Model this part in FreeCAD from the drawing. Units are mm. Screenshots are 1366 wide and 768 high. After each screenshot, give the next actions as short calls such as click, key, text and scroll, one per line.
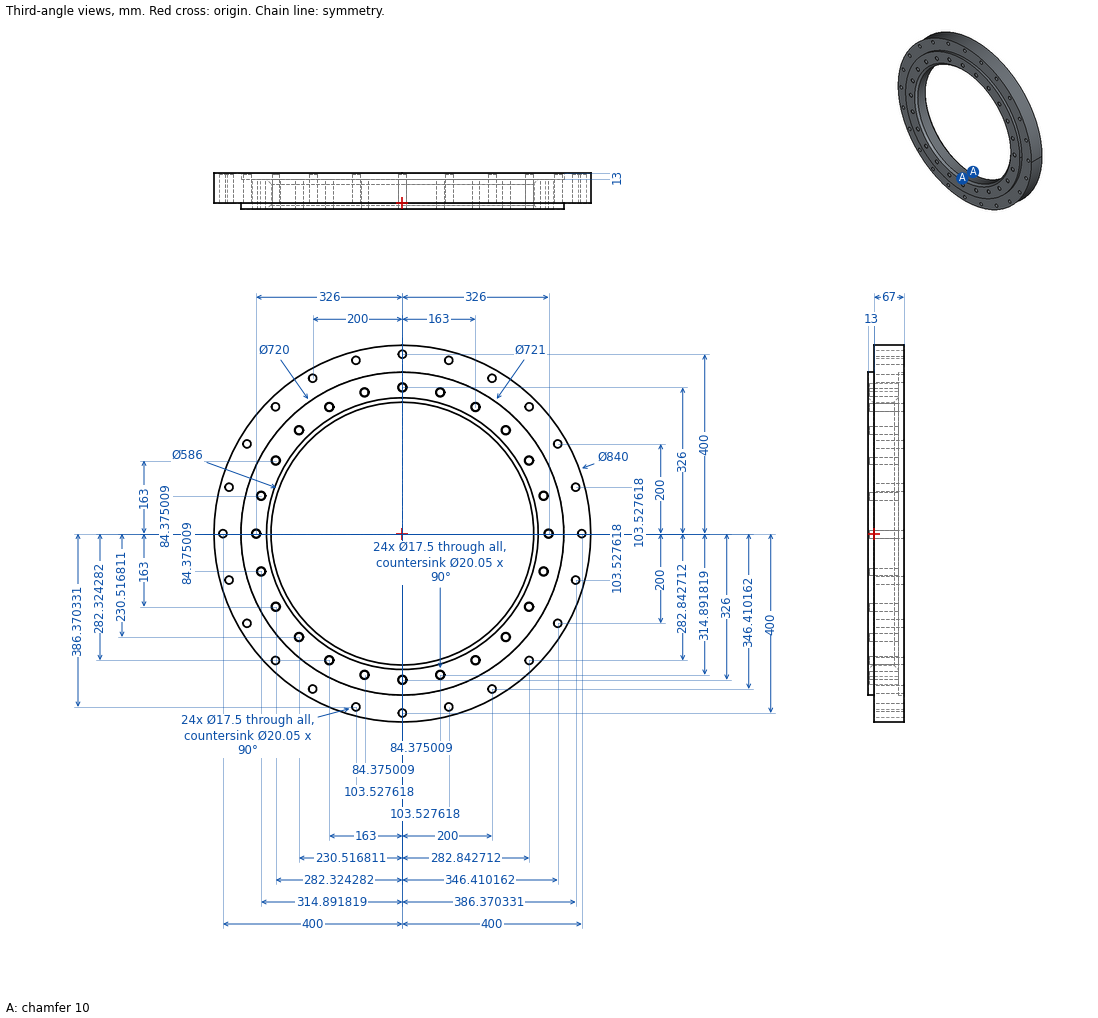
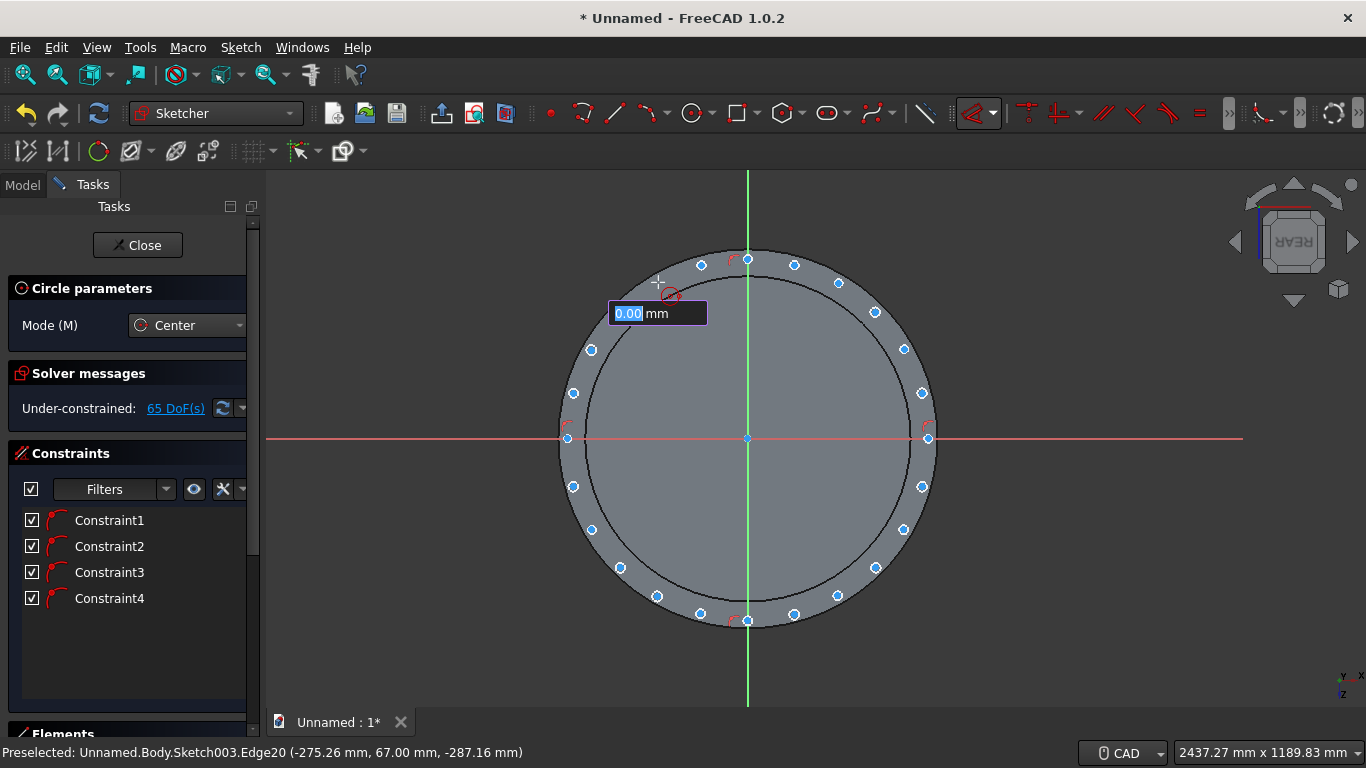
scroll(660, 280, up, 7)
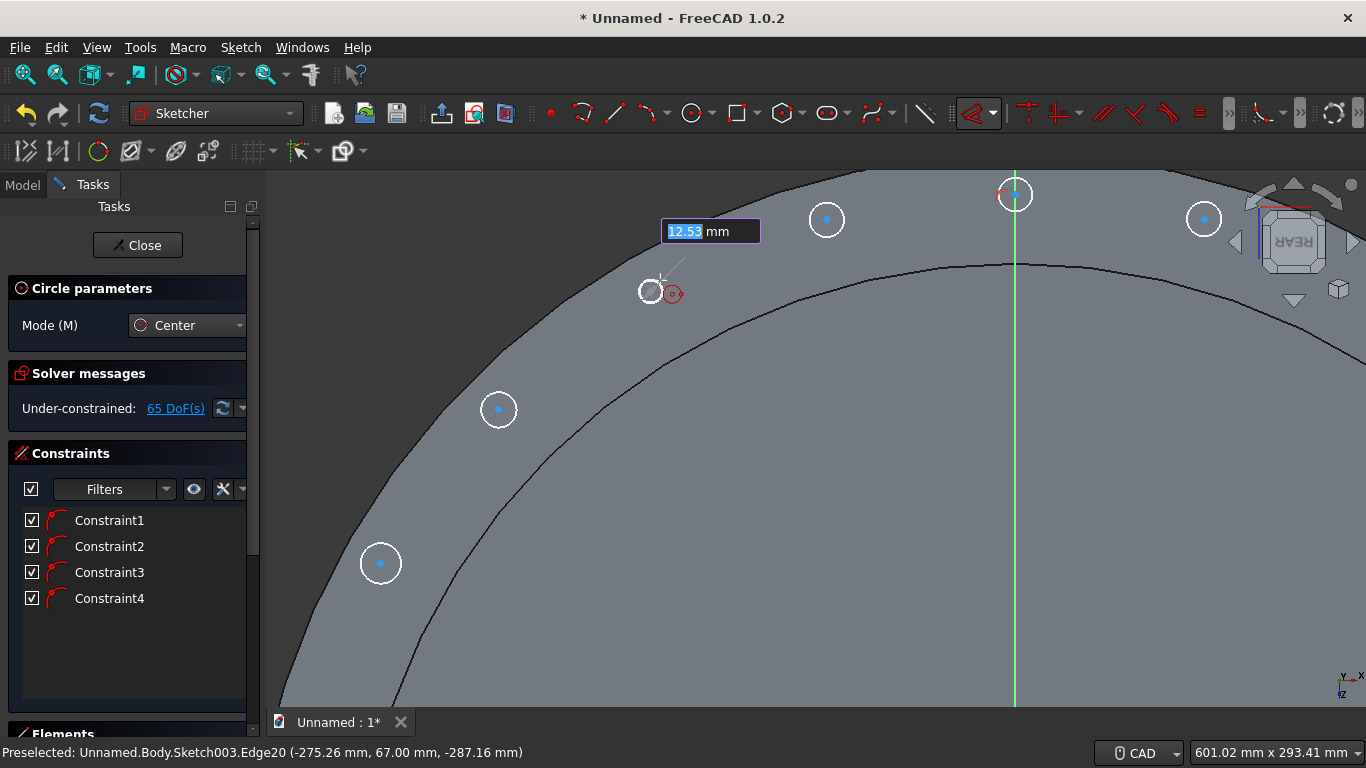
click(661, 278)
key(Escape)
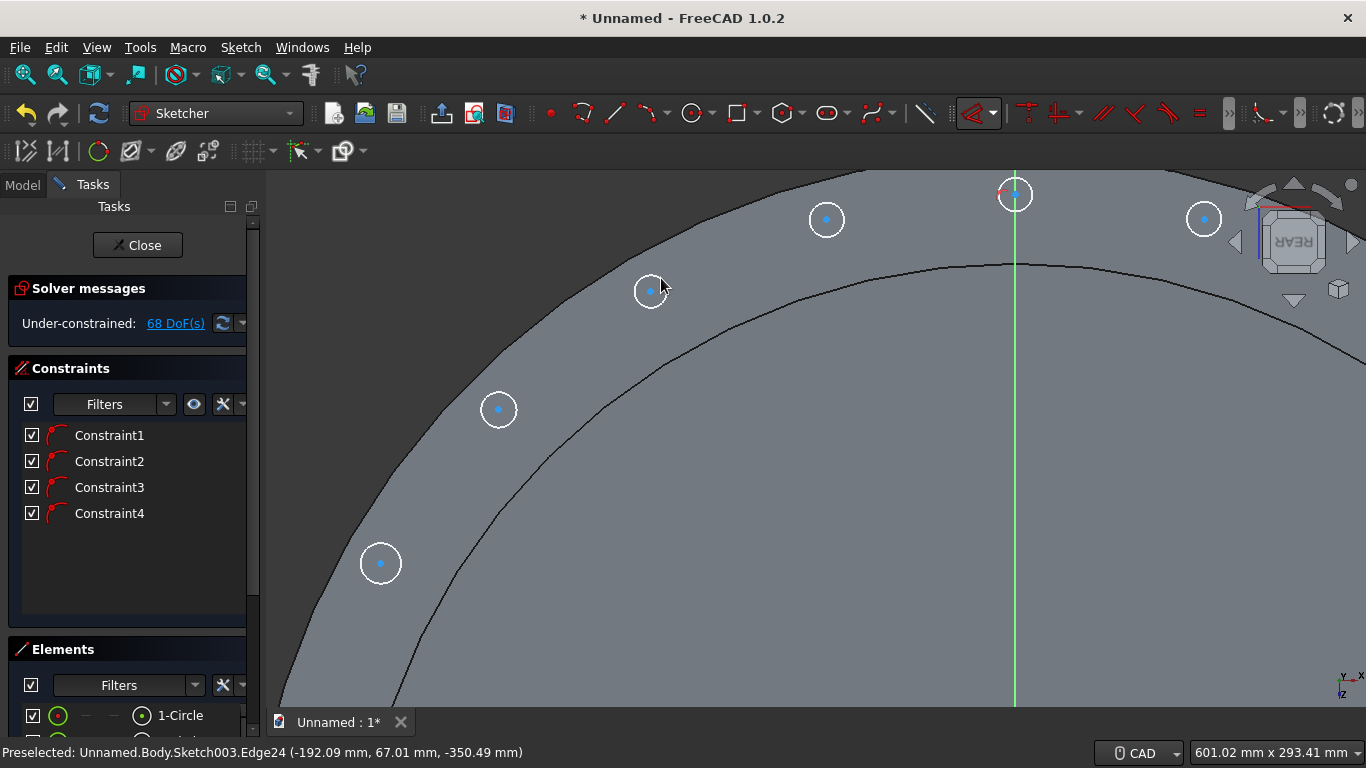
click(839, 208)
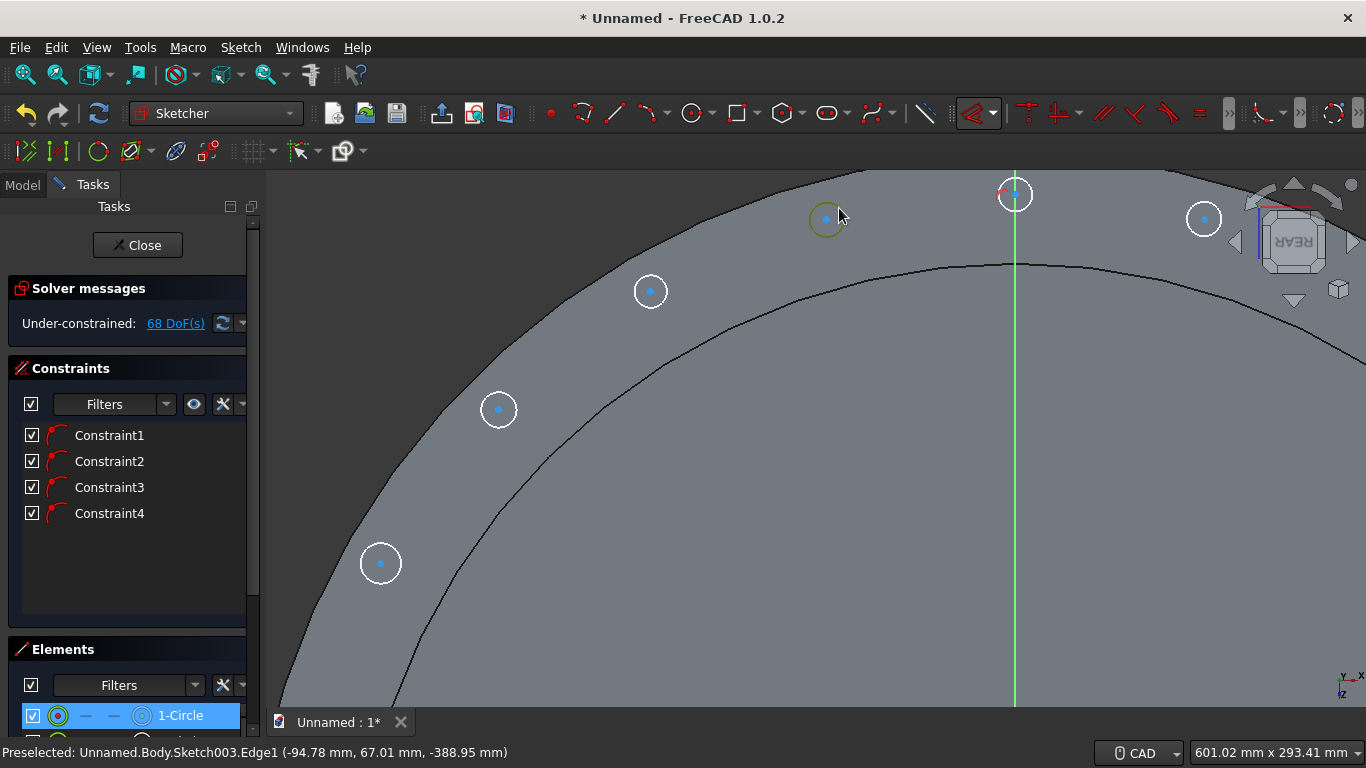
click(1004, 207)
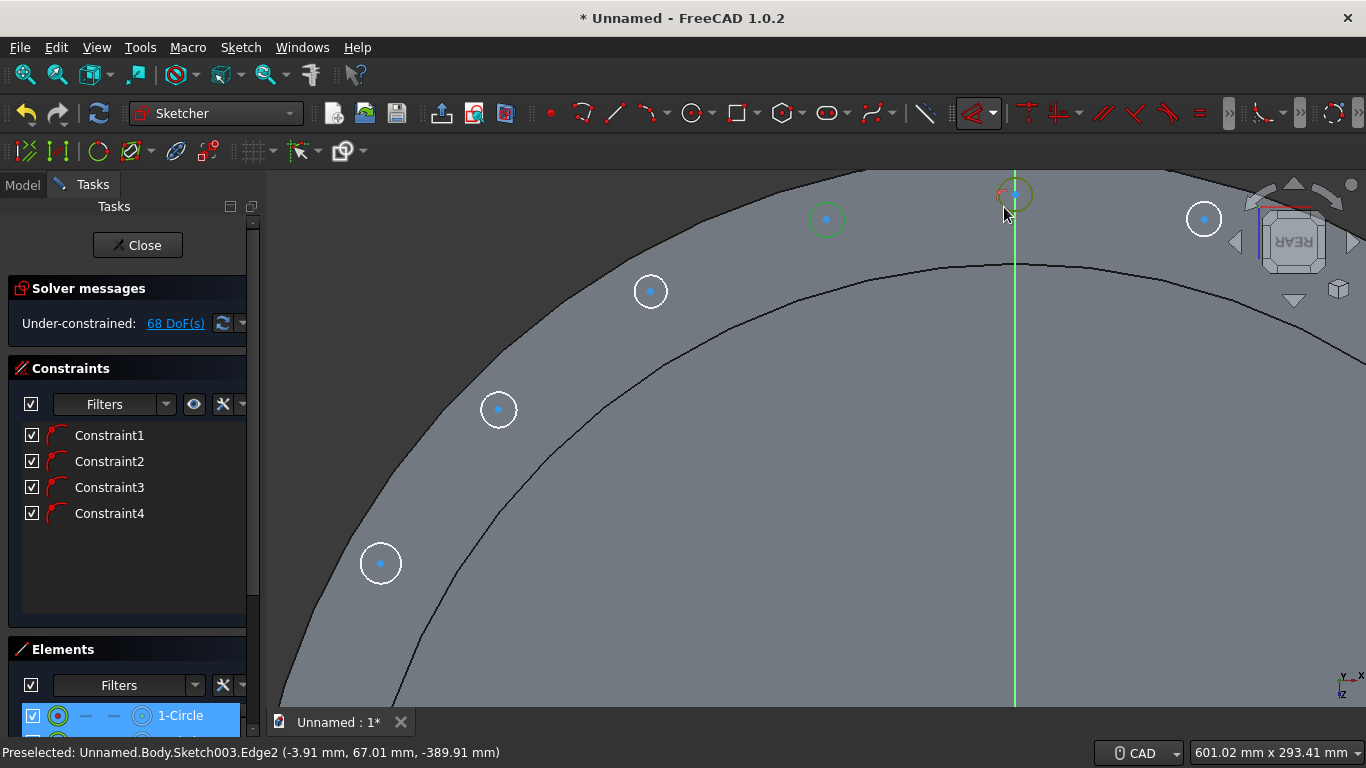
click(1192, 207)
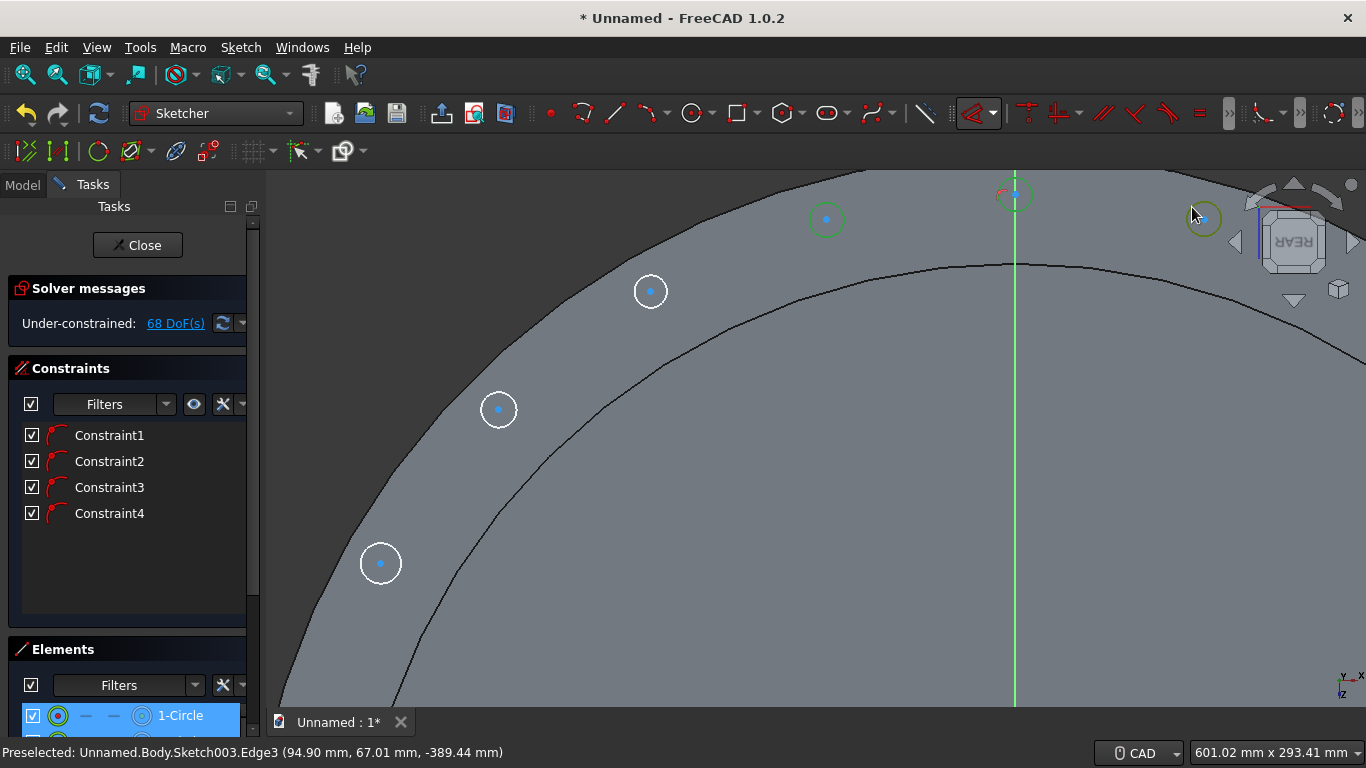
scroll(660, 280, down, 7)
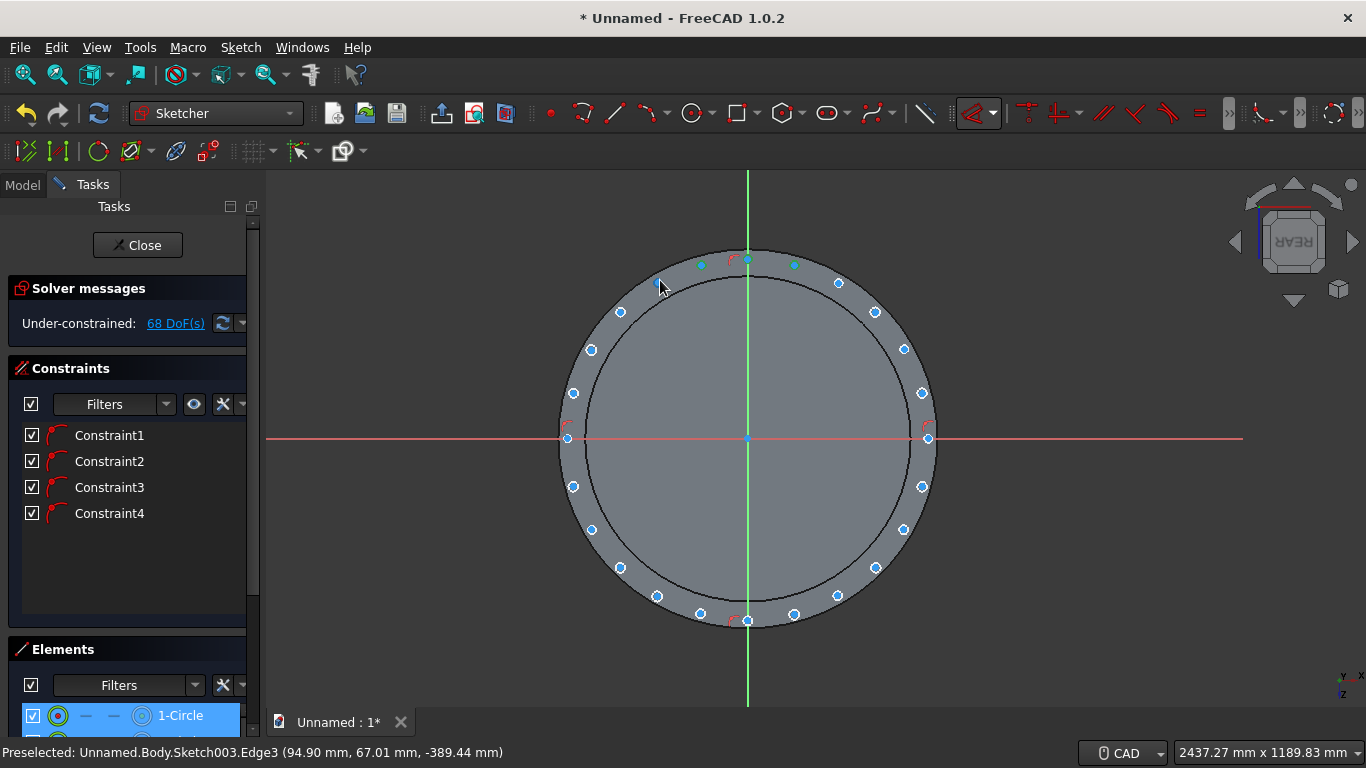
scroll(841, 280, up, 7)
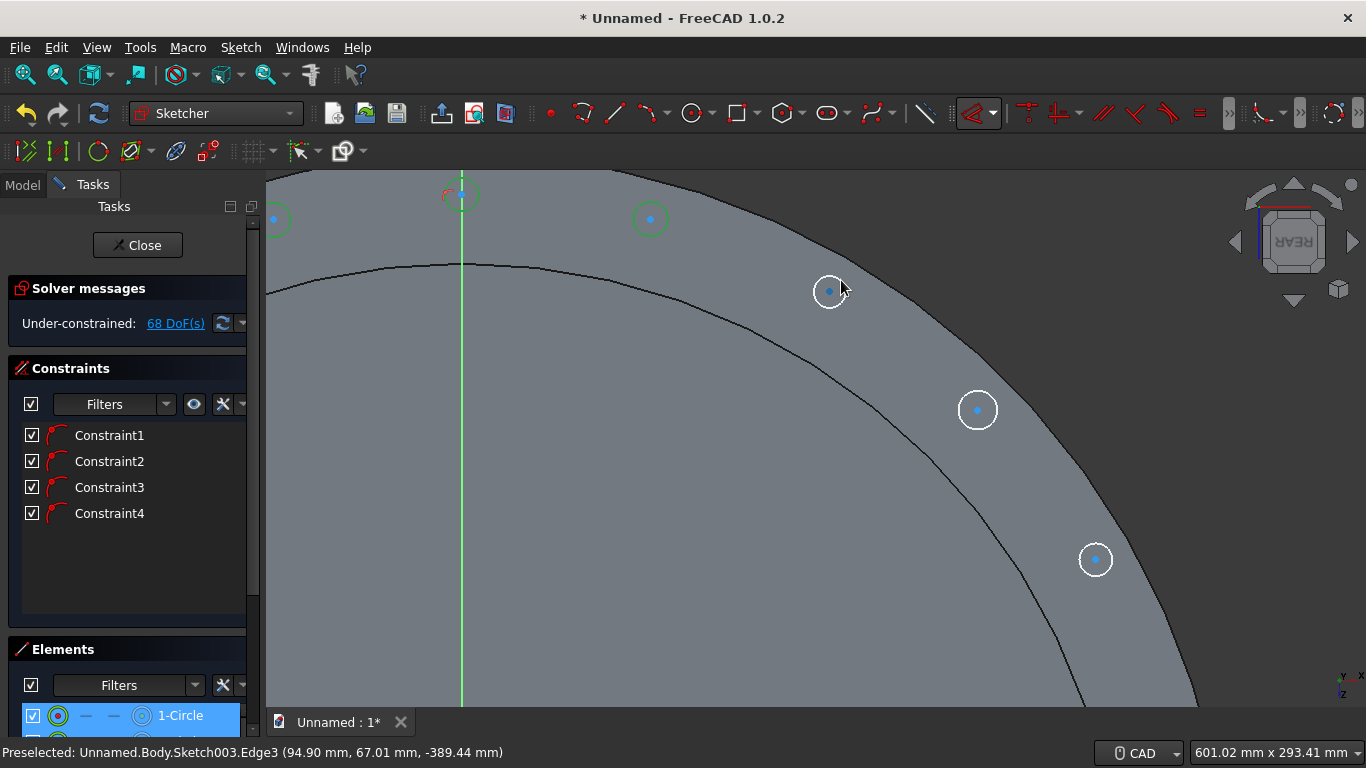
click(841, 281)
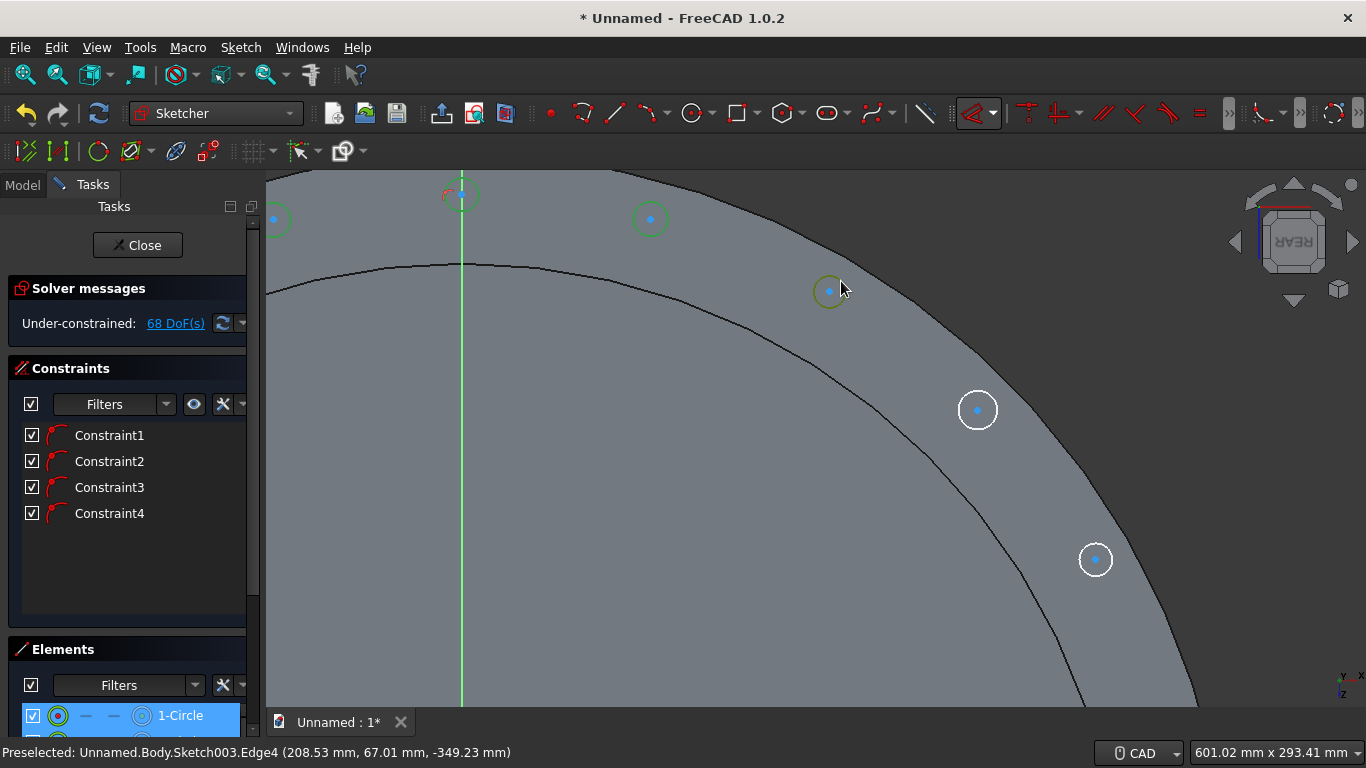
click(991, 396)